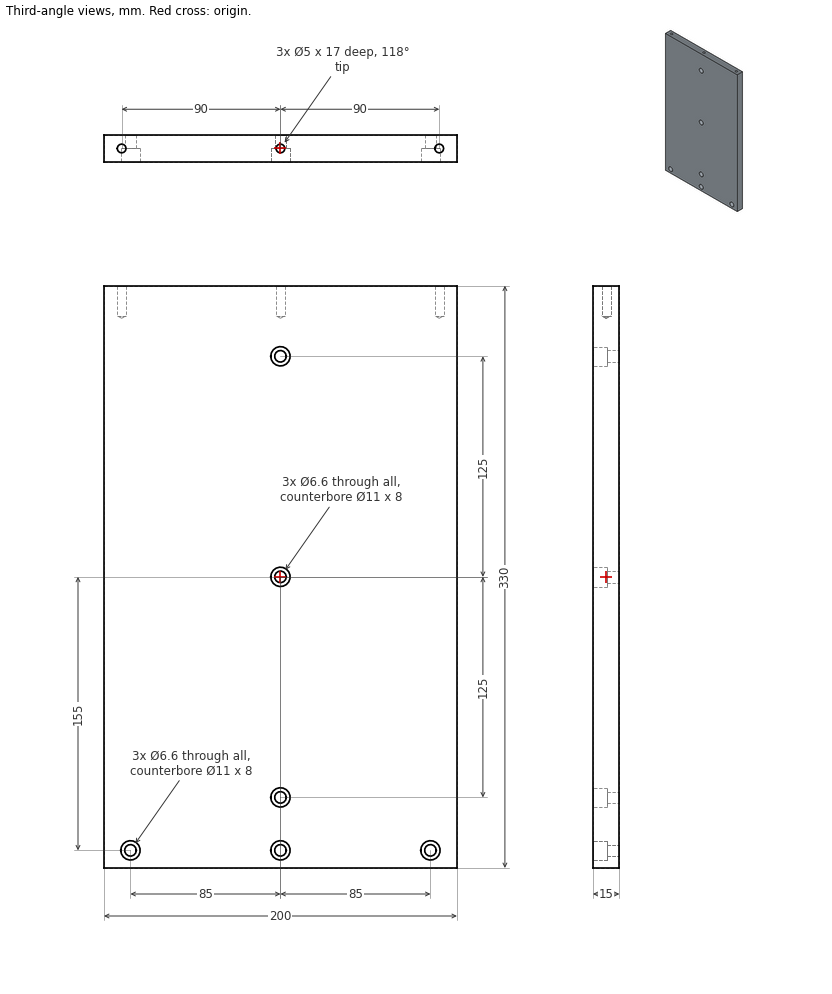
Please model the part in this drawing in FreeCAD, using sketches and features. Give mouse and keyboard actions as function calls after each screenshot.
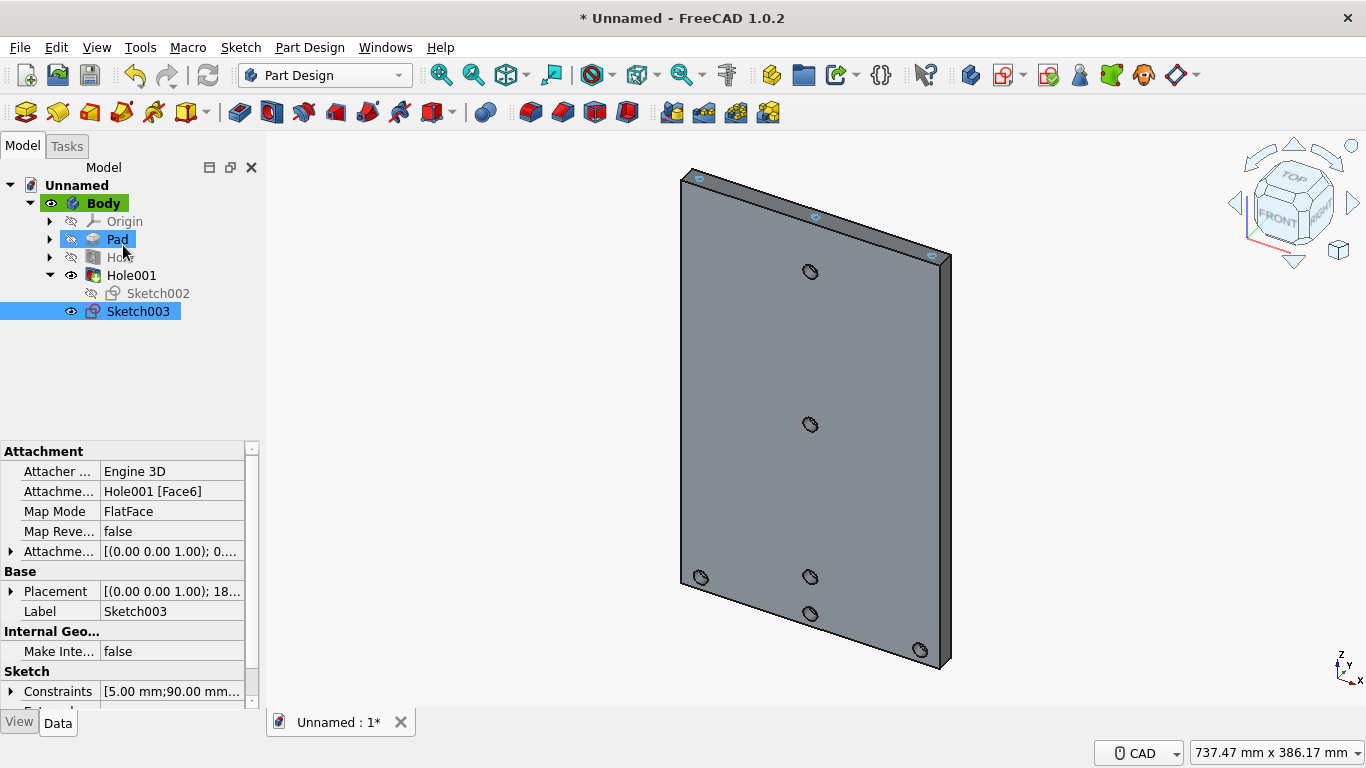
click(272, 112)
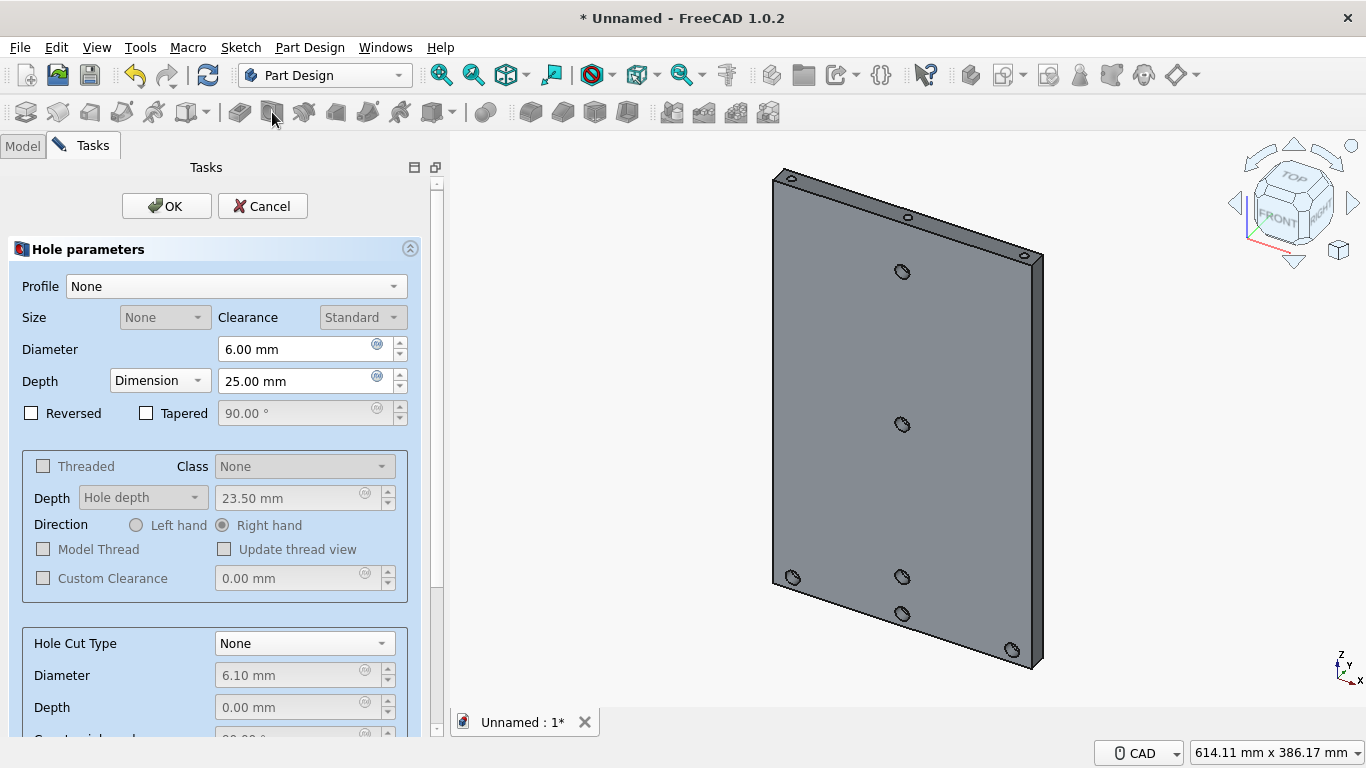
triple_click(305, 349)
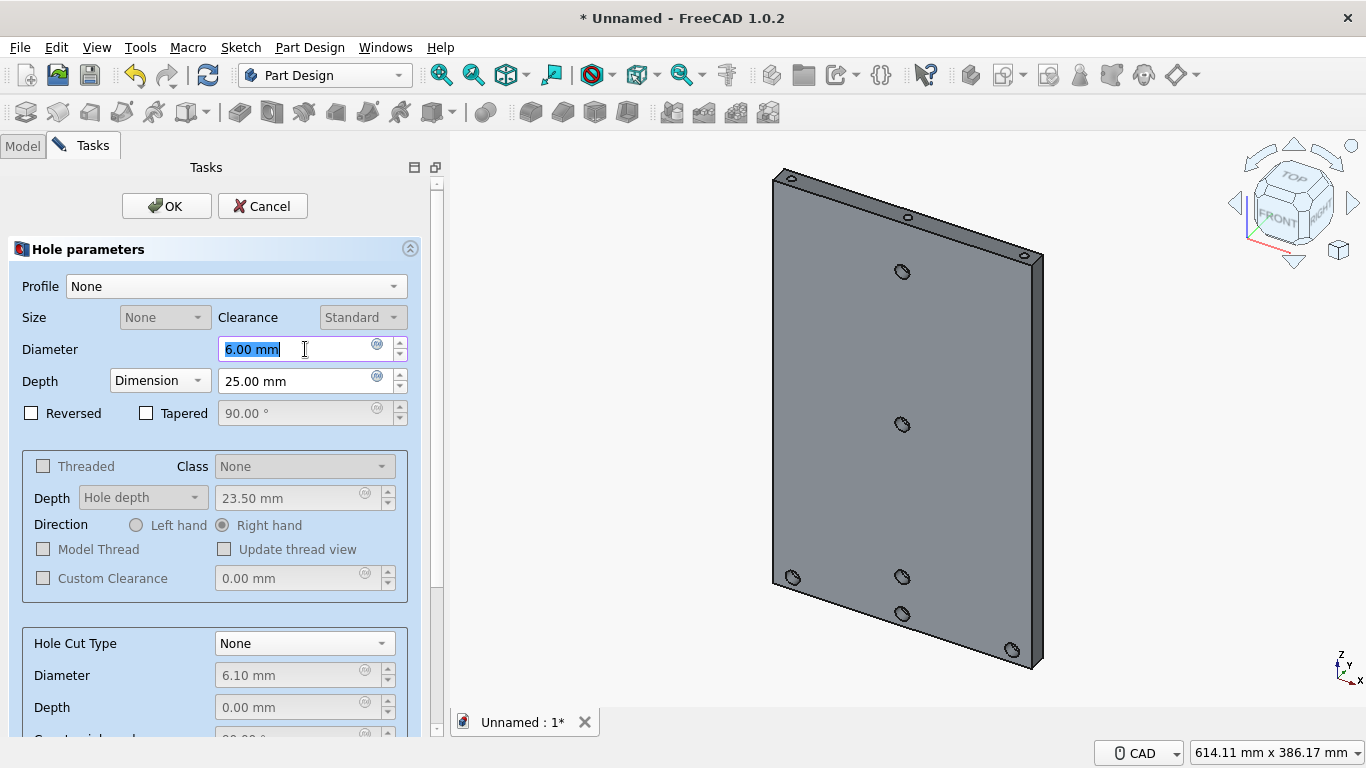
text(5)
key(Tab)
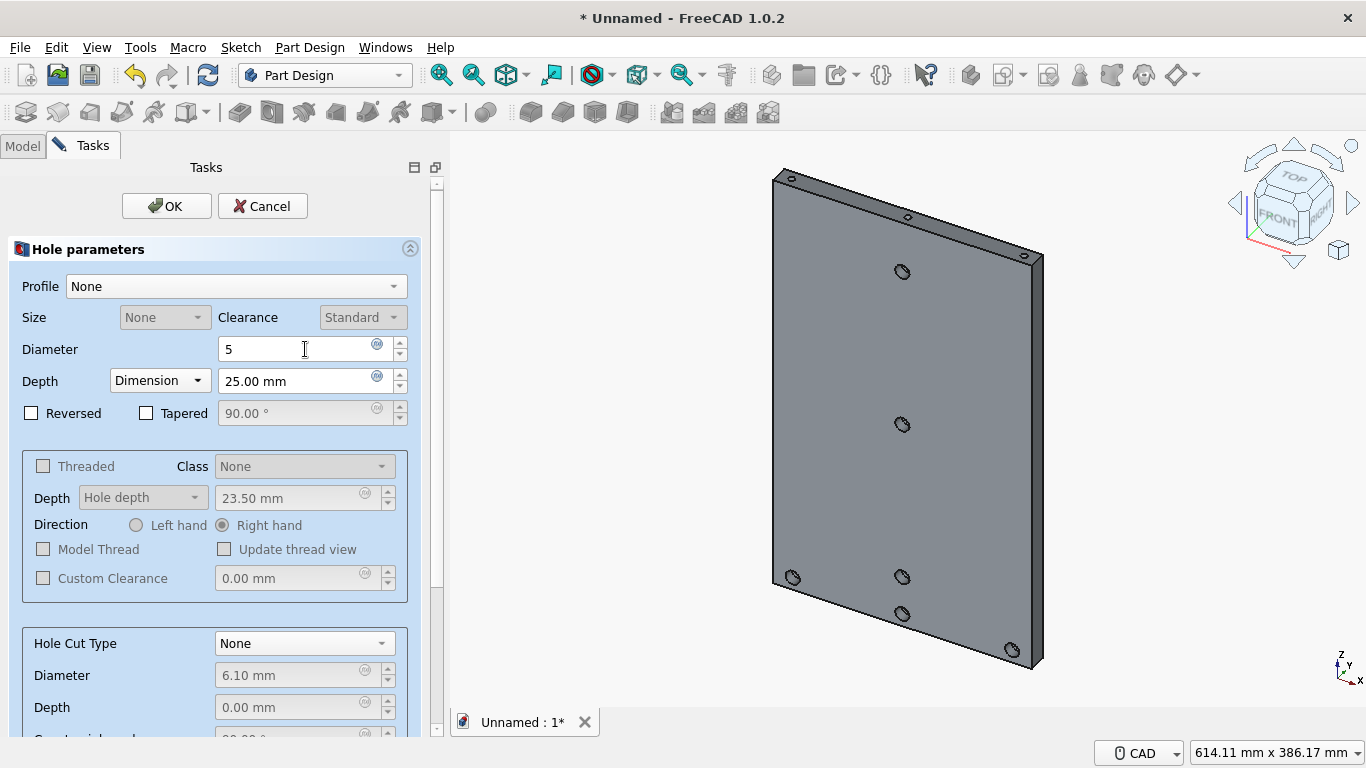
triple_click(305, 381)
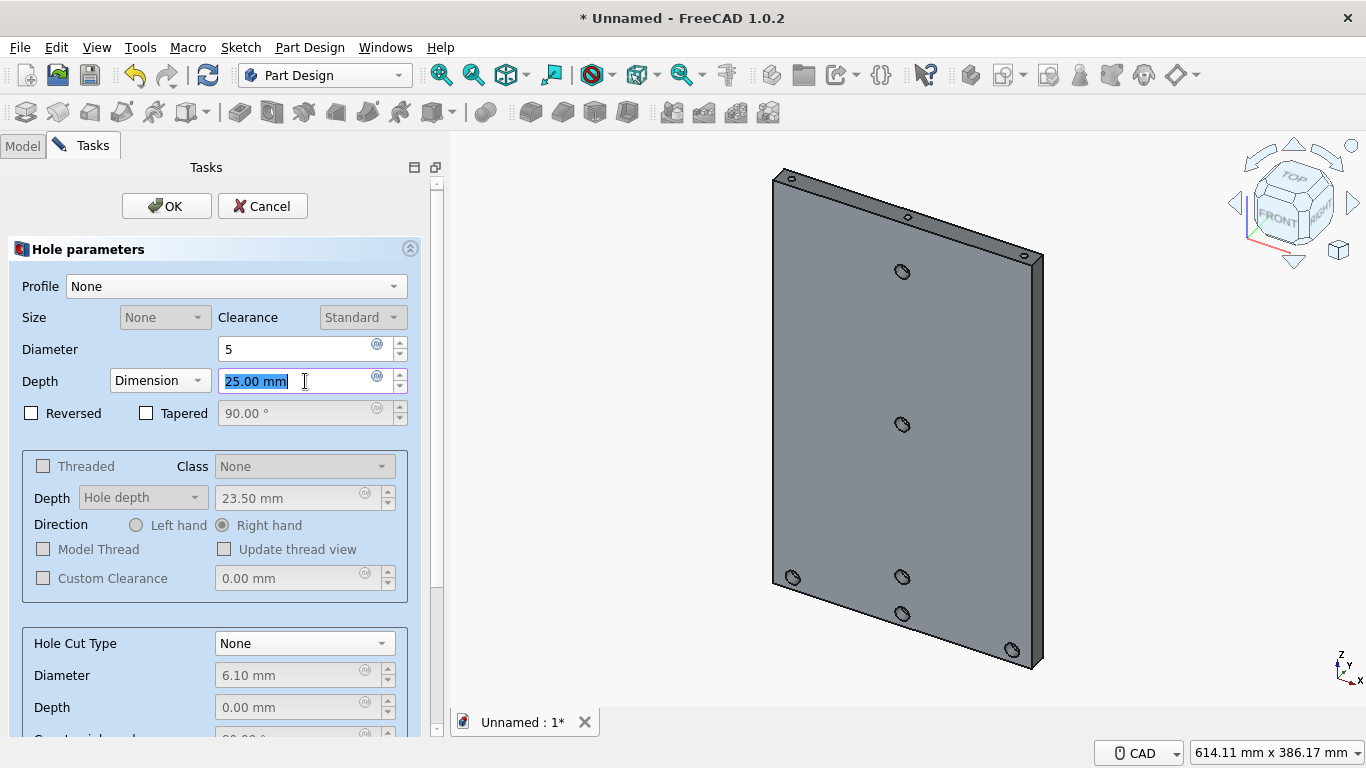
text(17)
key(Tab)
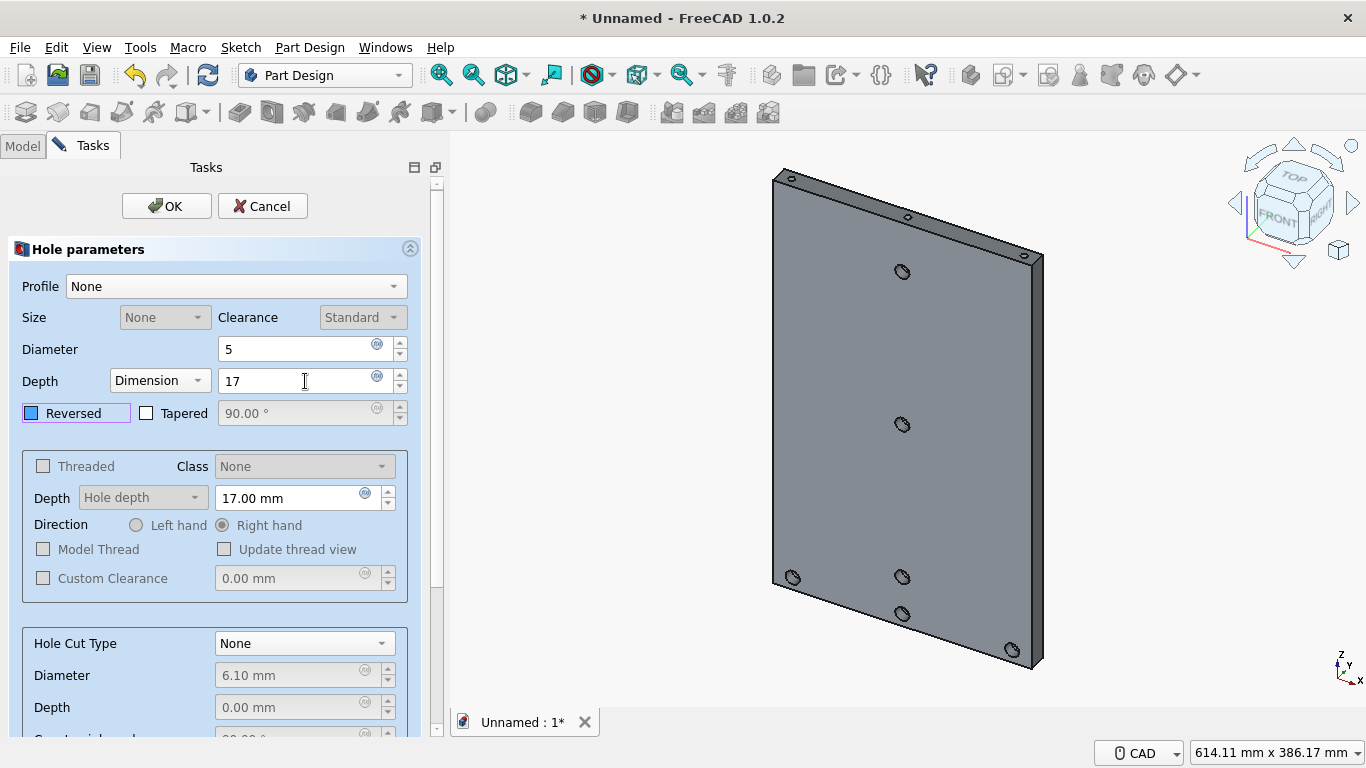
click(167, 206)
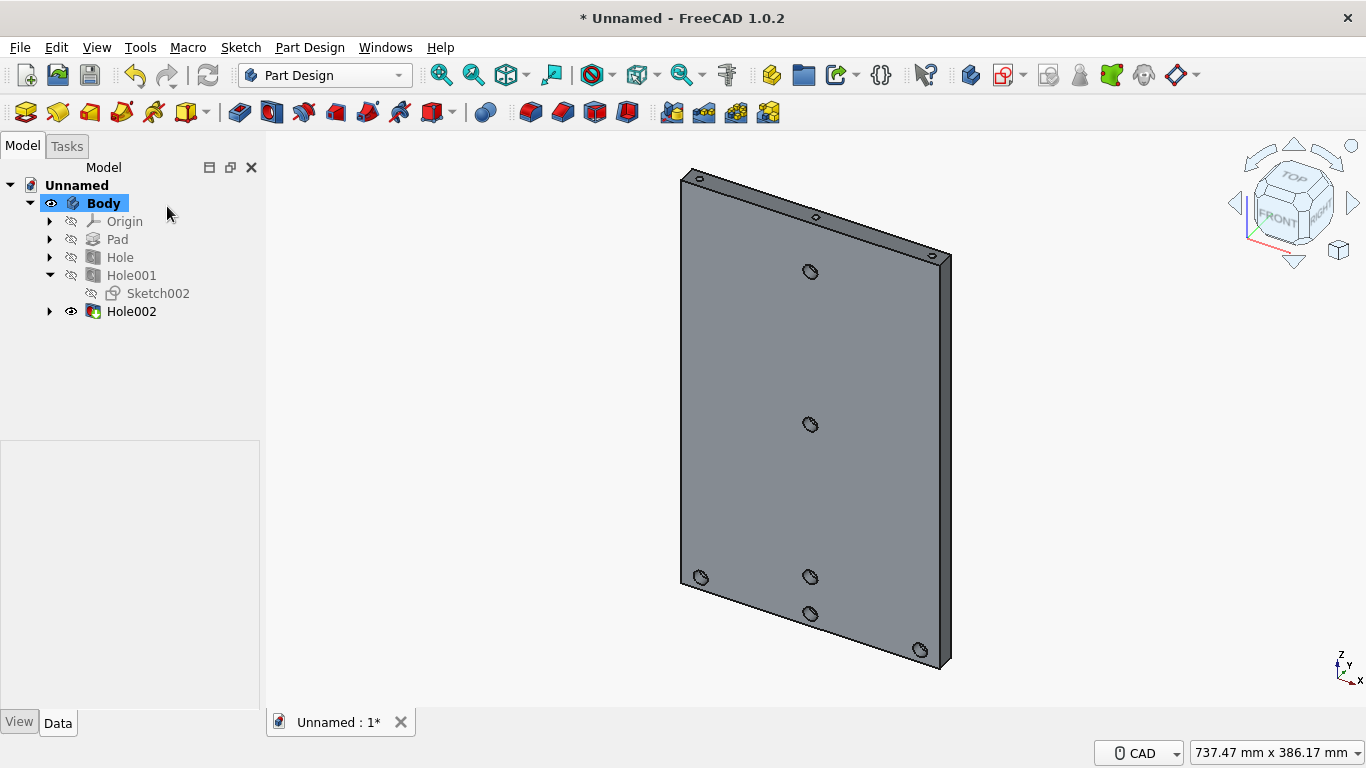
key(0)